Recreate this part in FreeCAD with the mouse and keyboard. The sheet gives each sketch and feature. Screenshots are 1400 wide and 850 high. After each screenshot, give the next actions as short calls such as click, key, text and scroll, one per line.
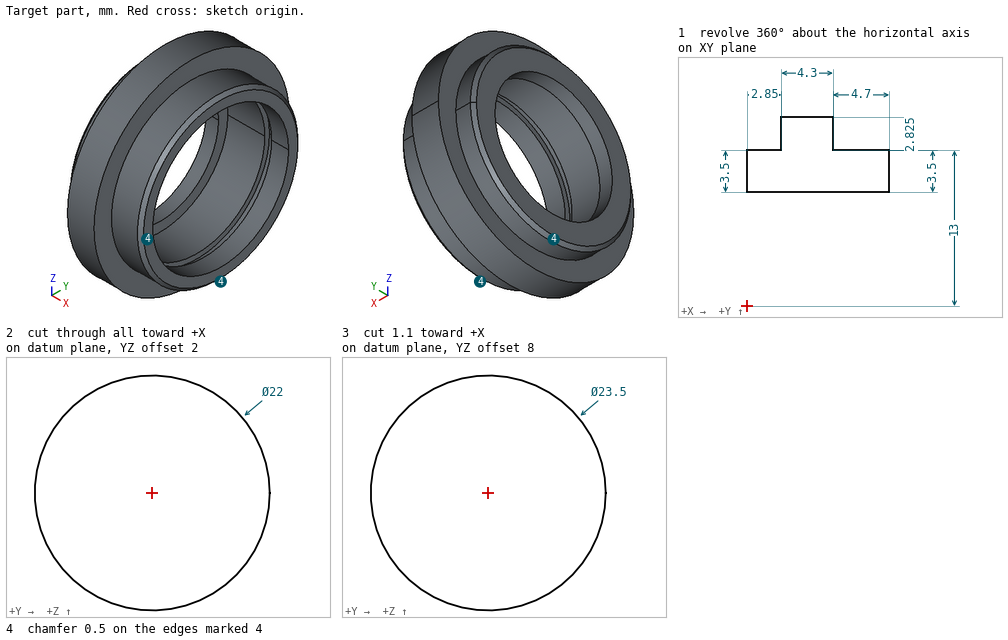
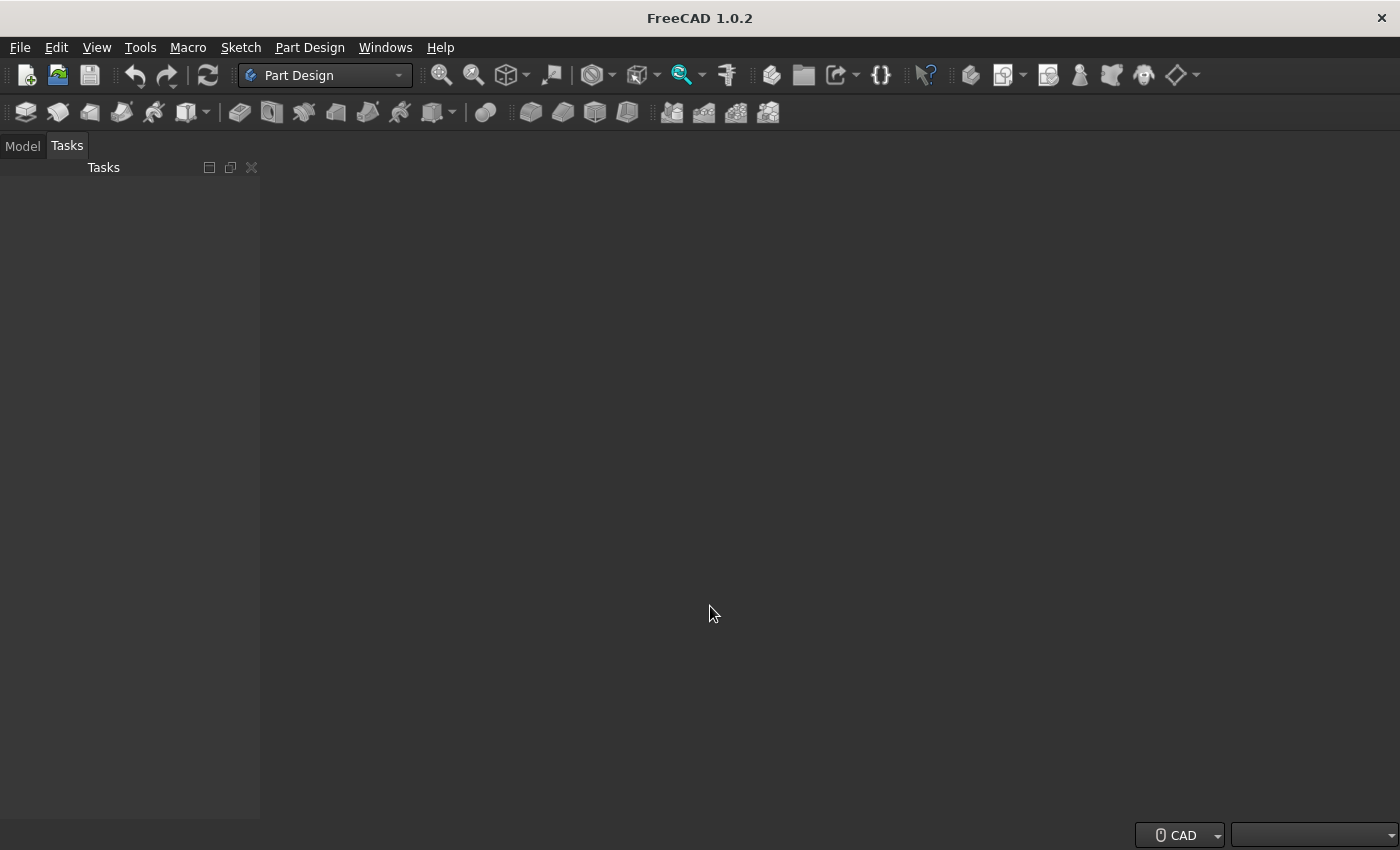
click(26, 76)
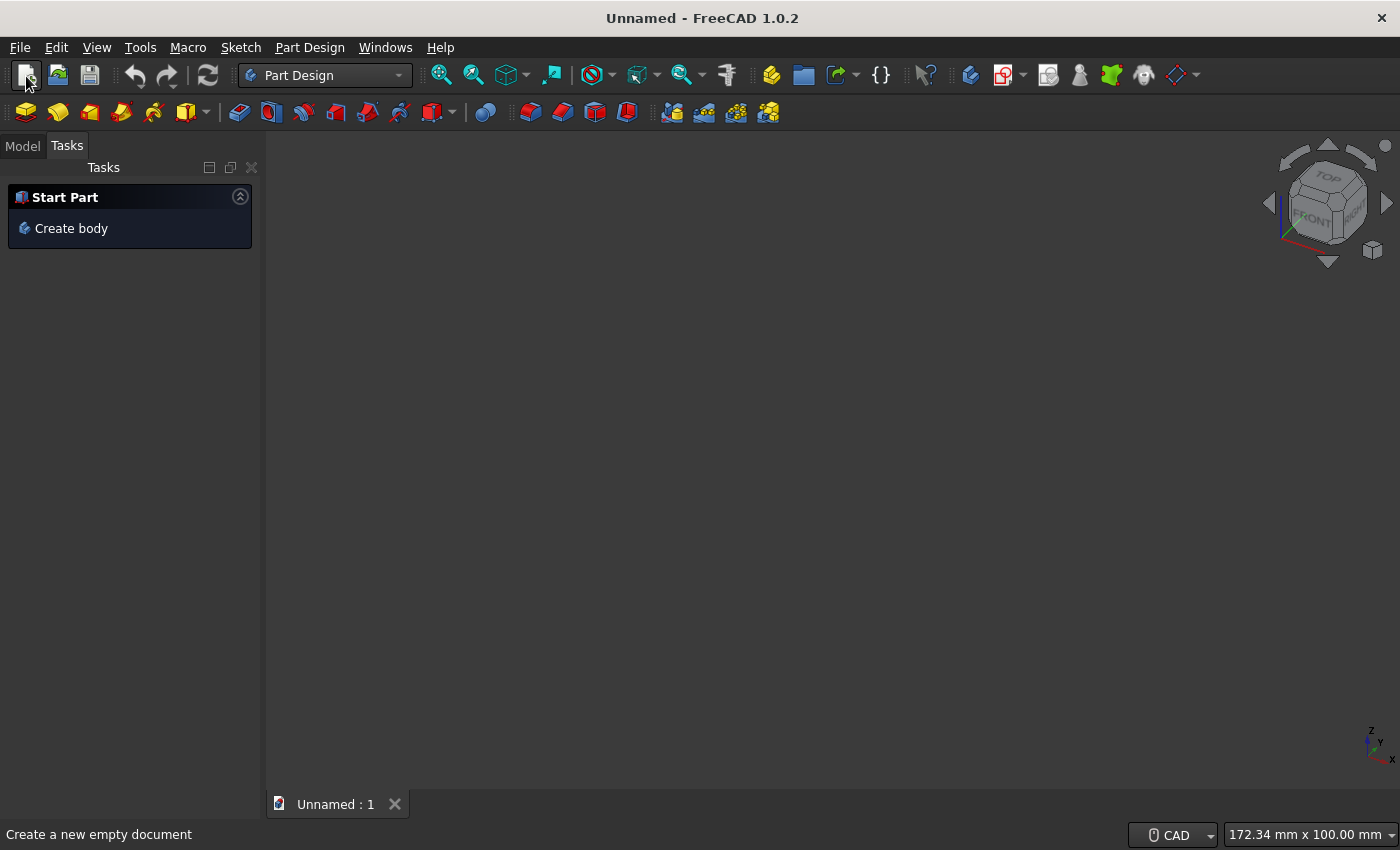
click(1004, 76)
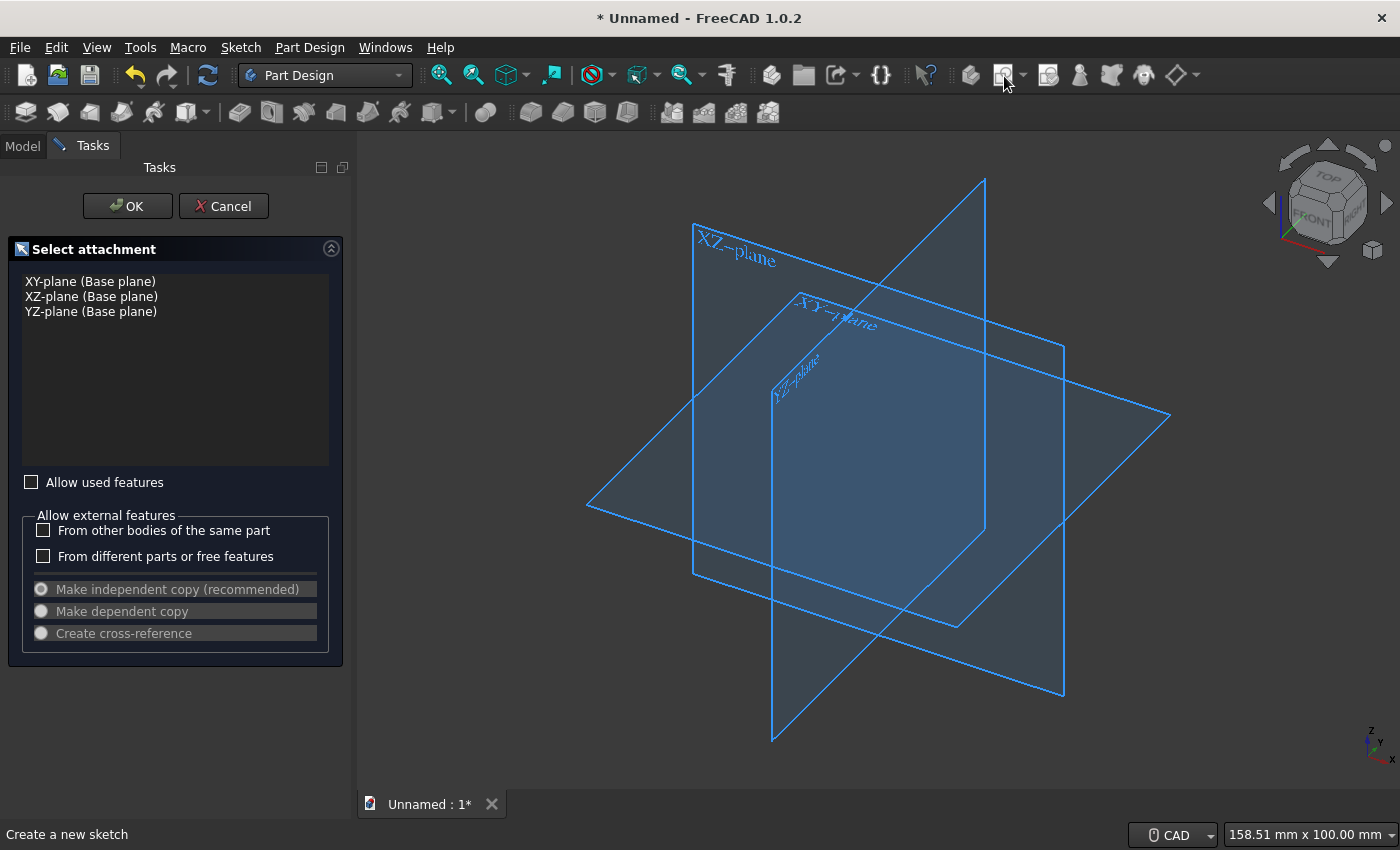
click(82, 282)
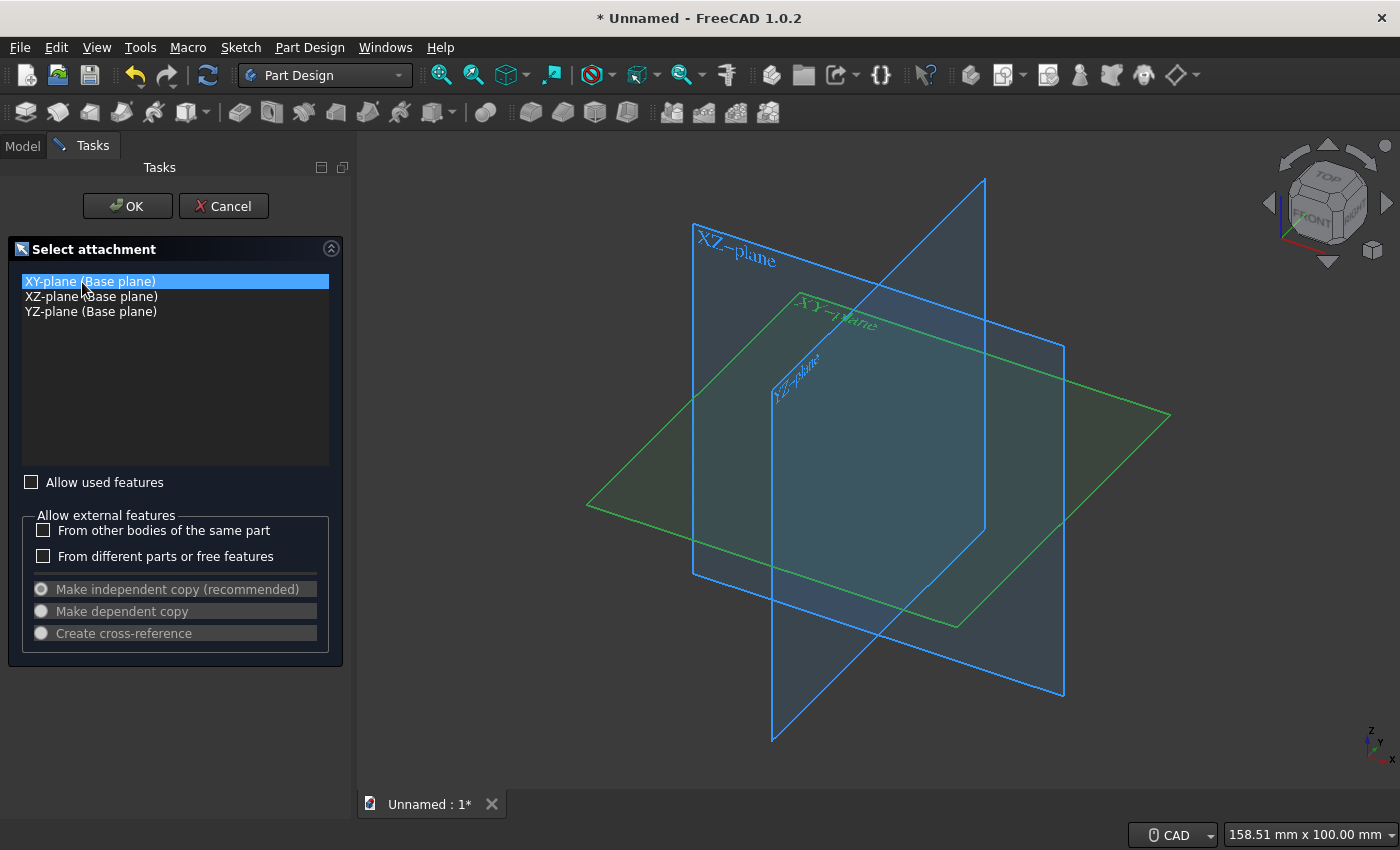
click(128, 206)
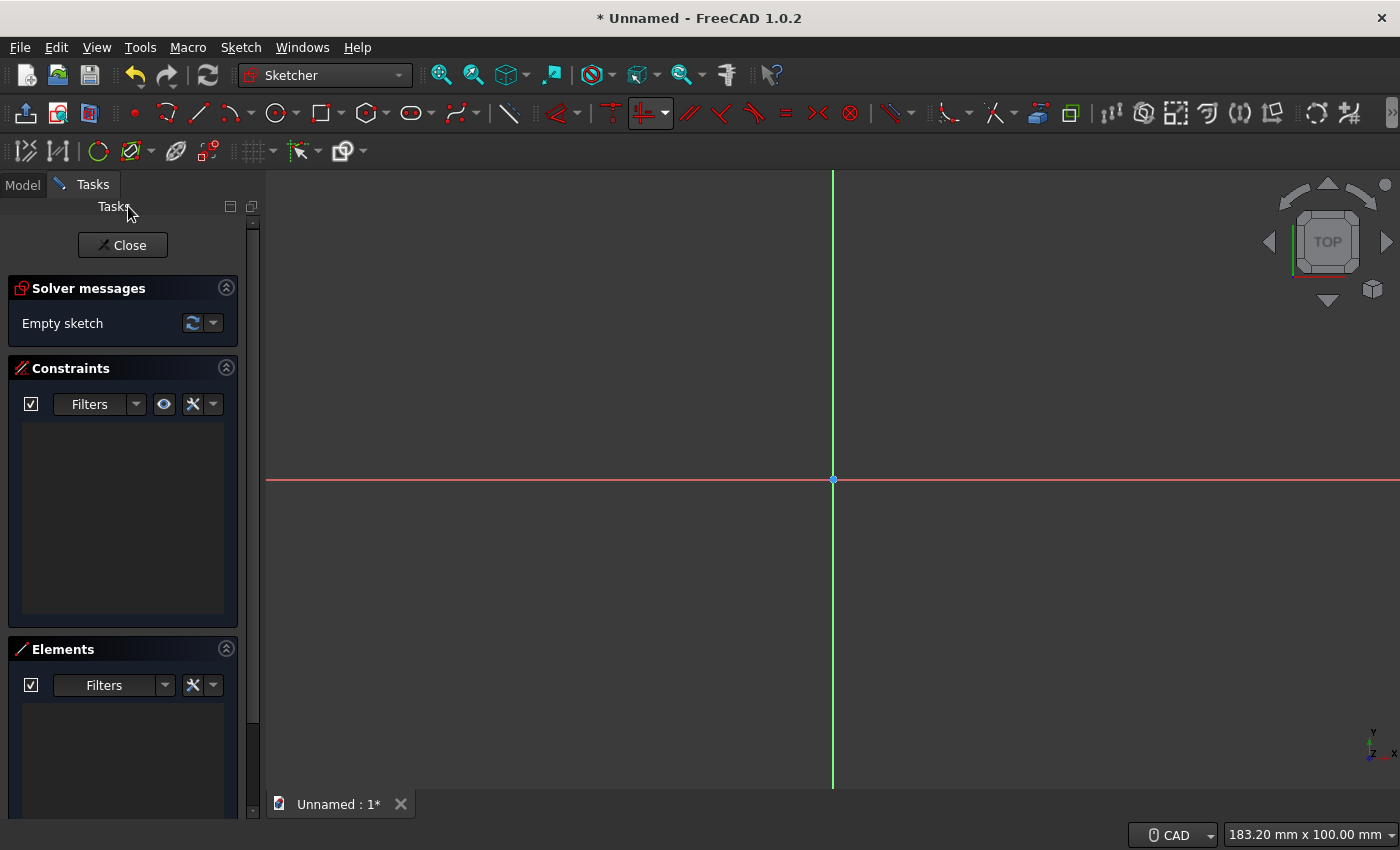
scroll(904, 414, up, 7)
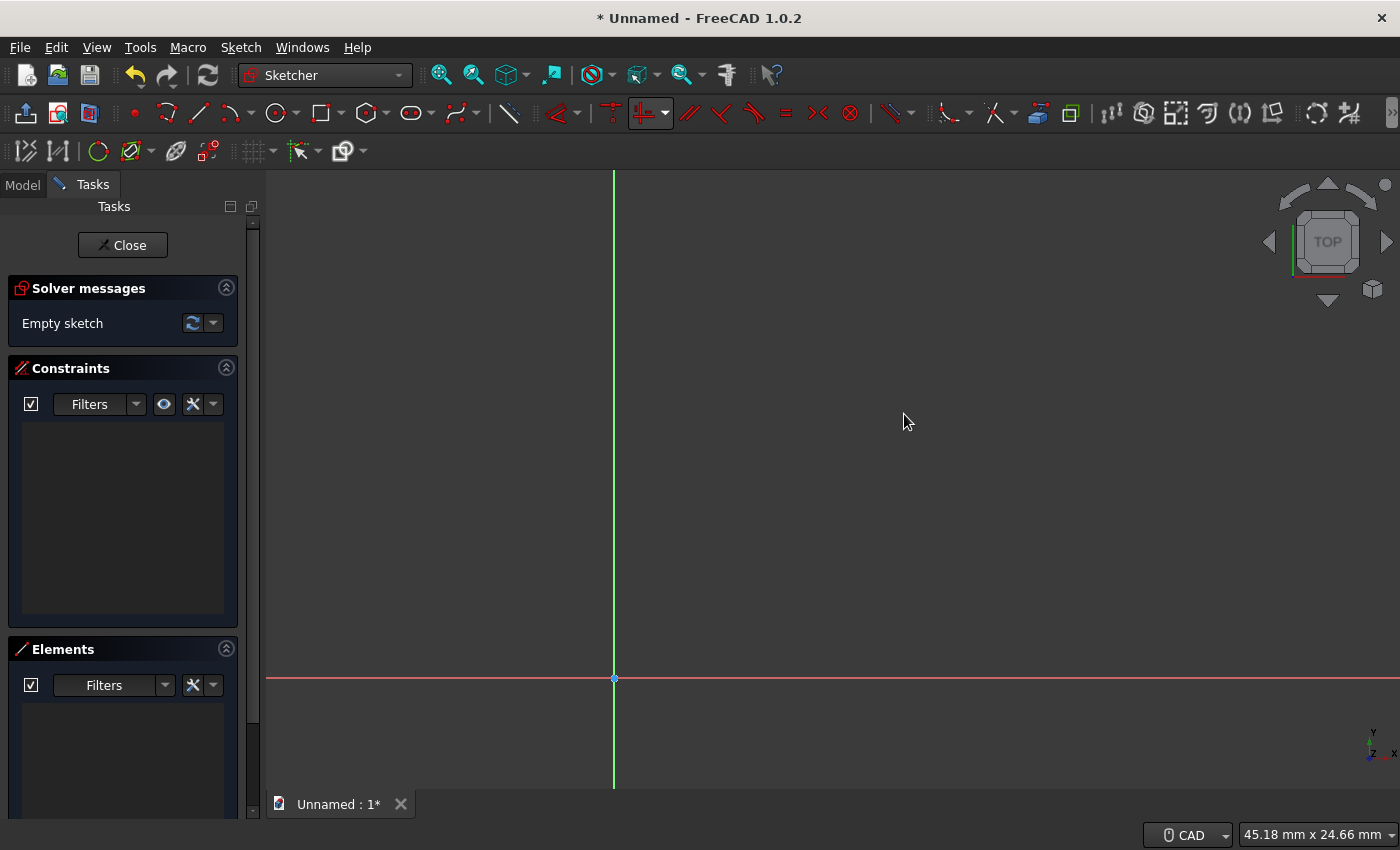
click(168, 114)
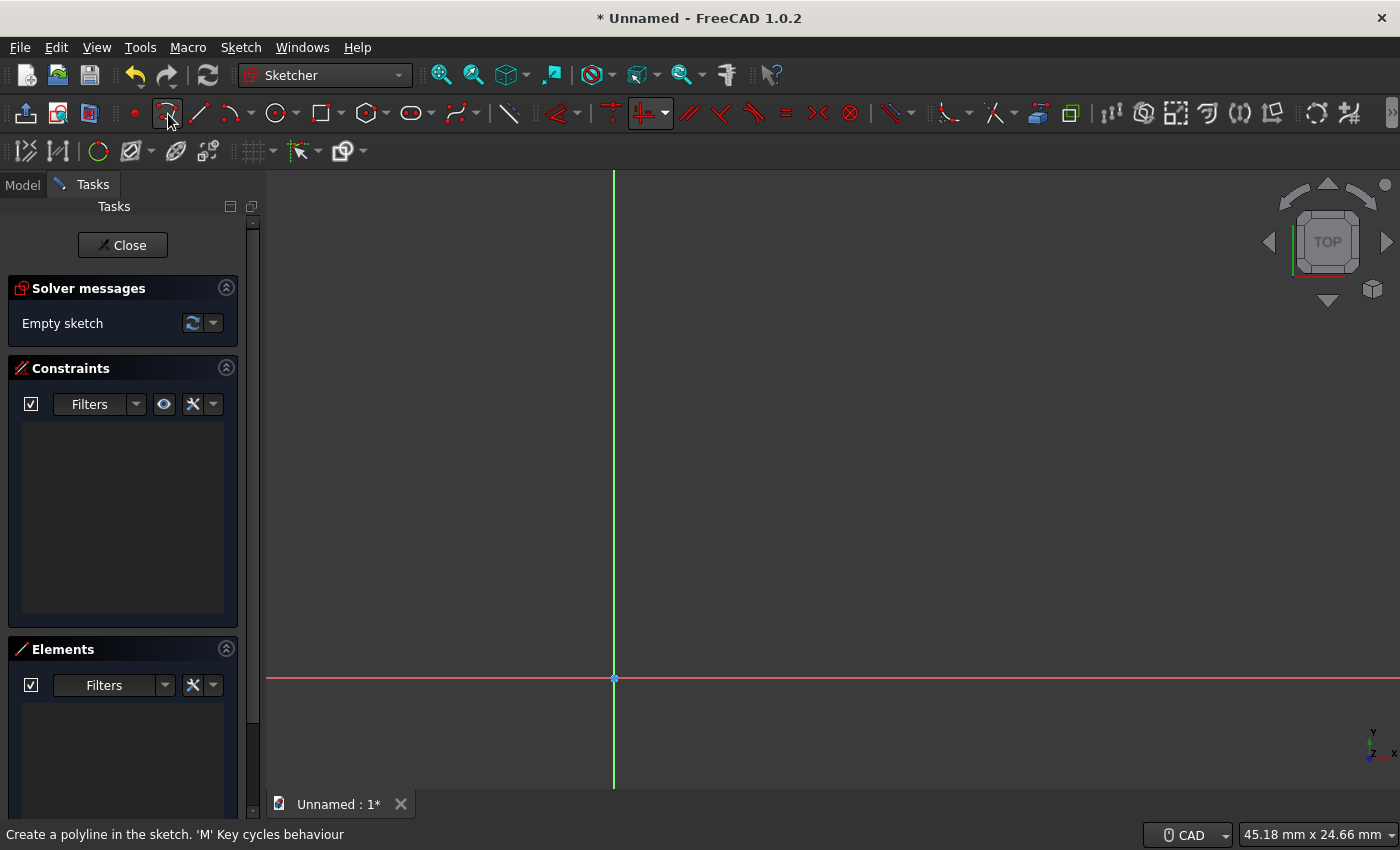
click(614, 440)
click(912, 440)
click(912, 352)
click(794, 352)
click(794, 281)
click(686, 281)
click(686, 352)
click(623, 352)
click(614, 441)
key(Escape)
key(Escape)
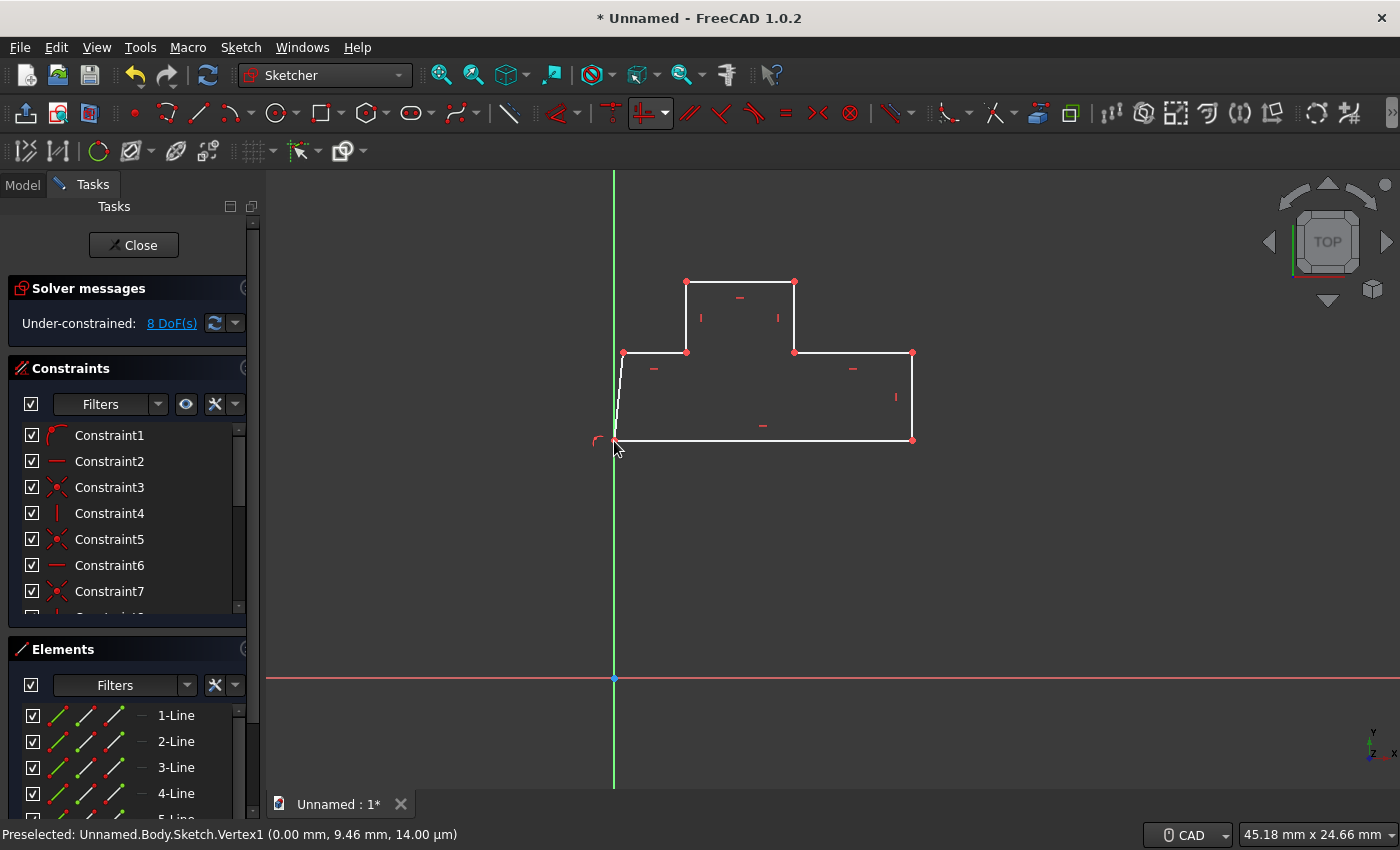
click(617, 415)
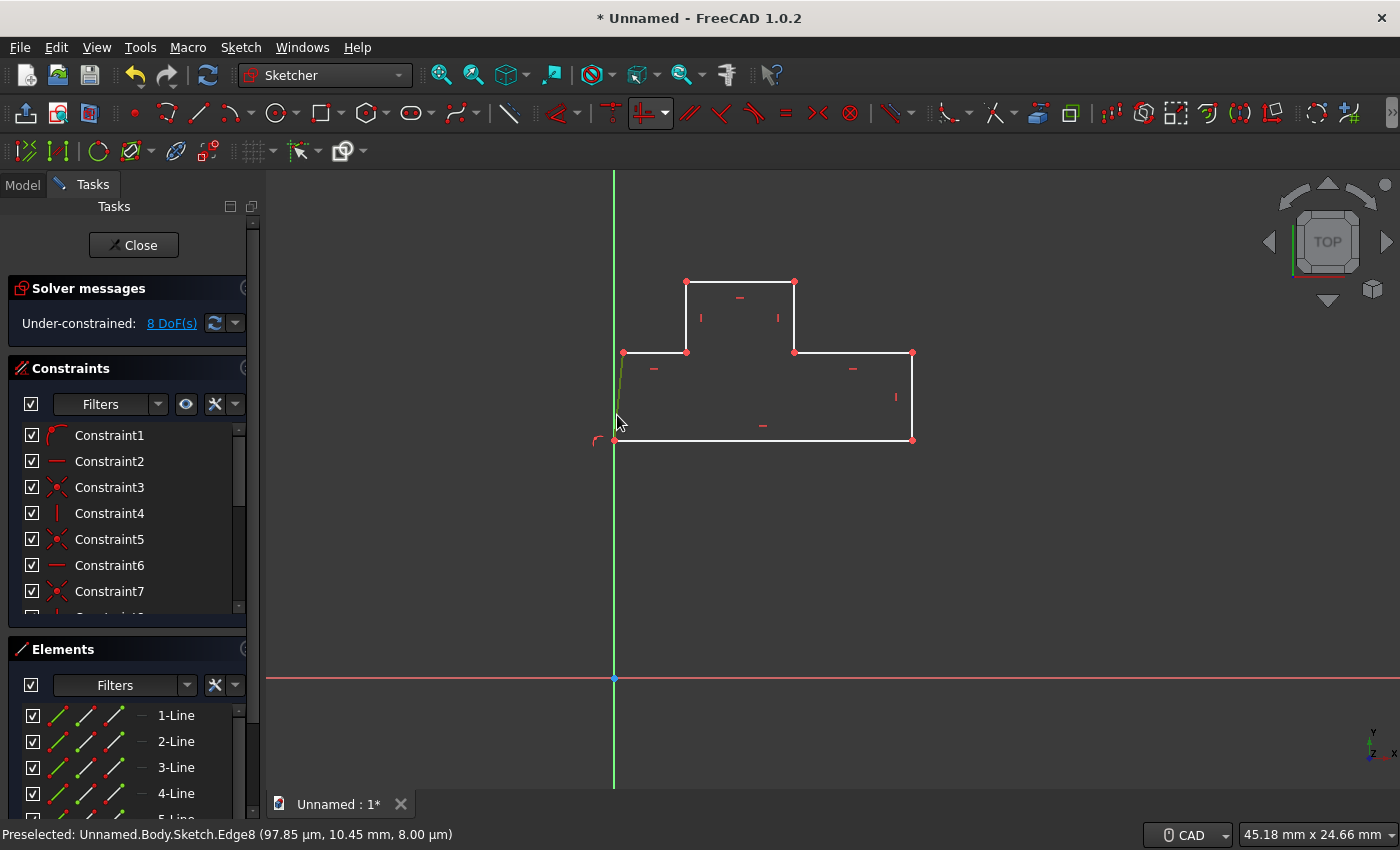
key(v)